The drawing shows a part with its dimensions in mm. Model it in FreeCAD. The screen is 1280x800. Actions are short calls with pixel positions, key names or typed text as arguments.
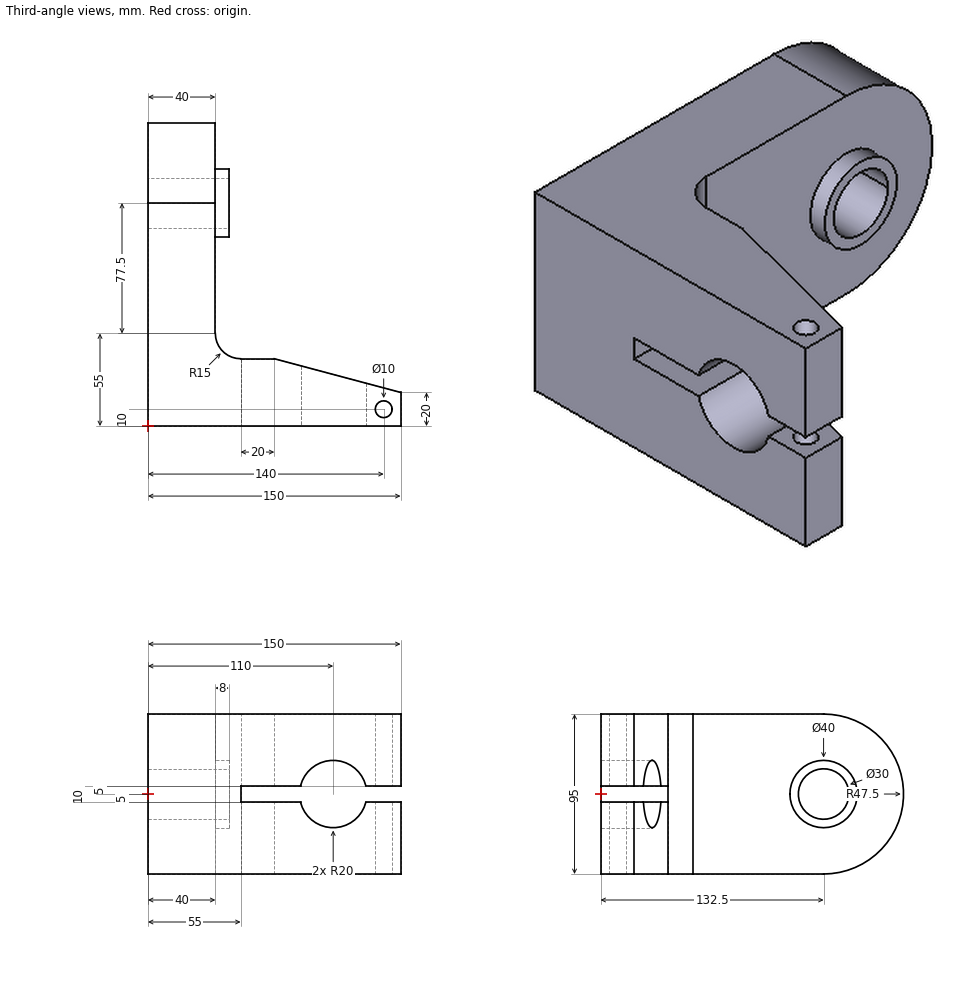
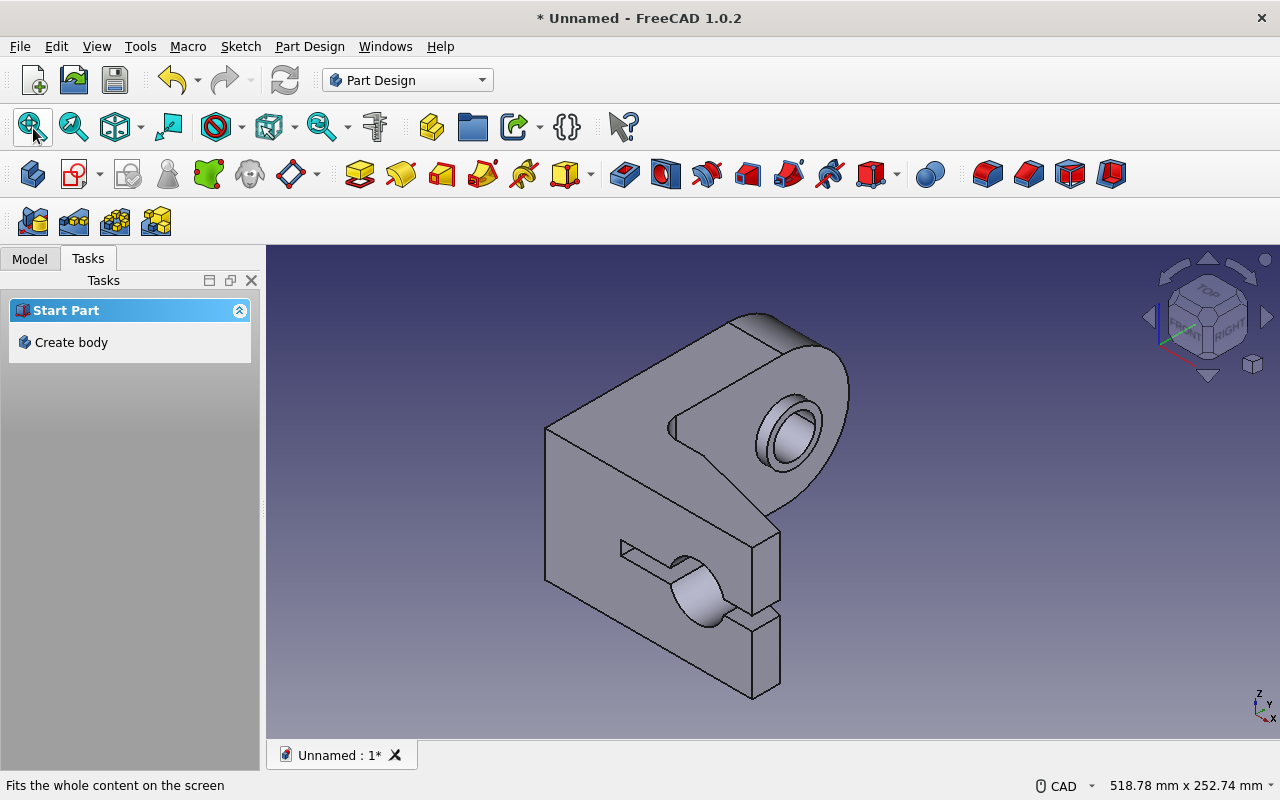
click(629, 430)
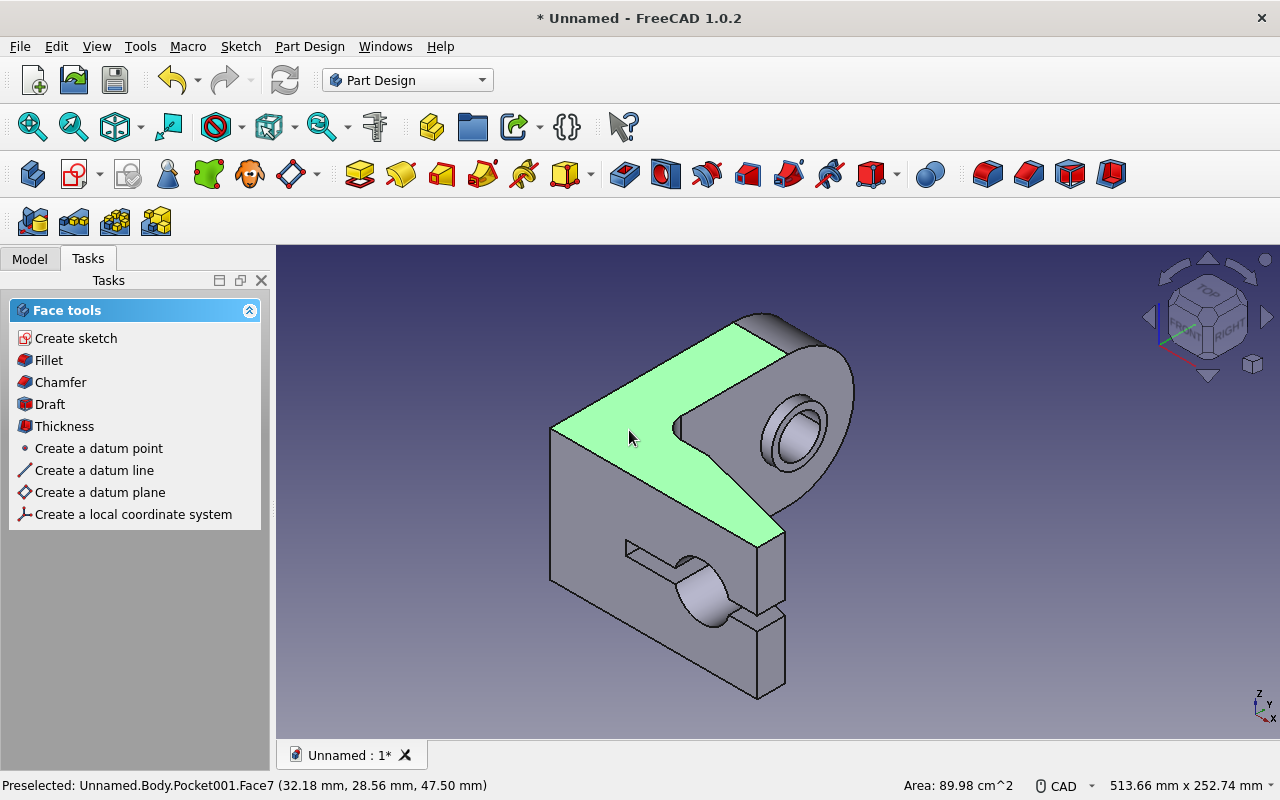
click(74, 174)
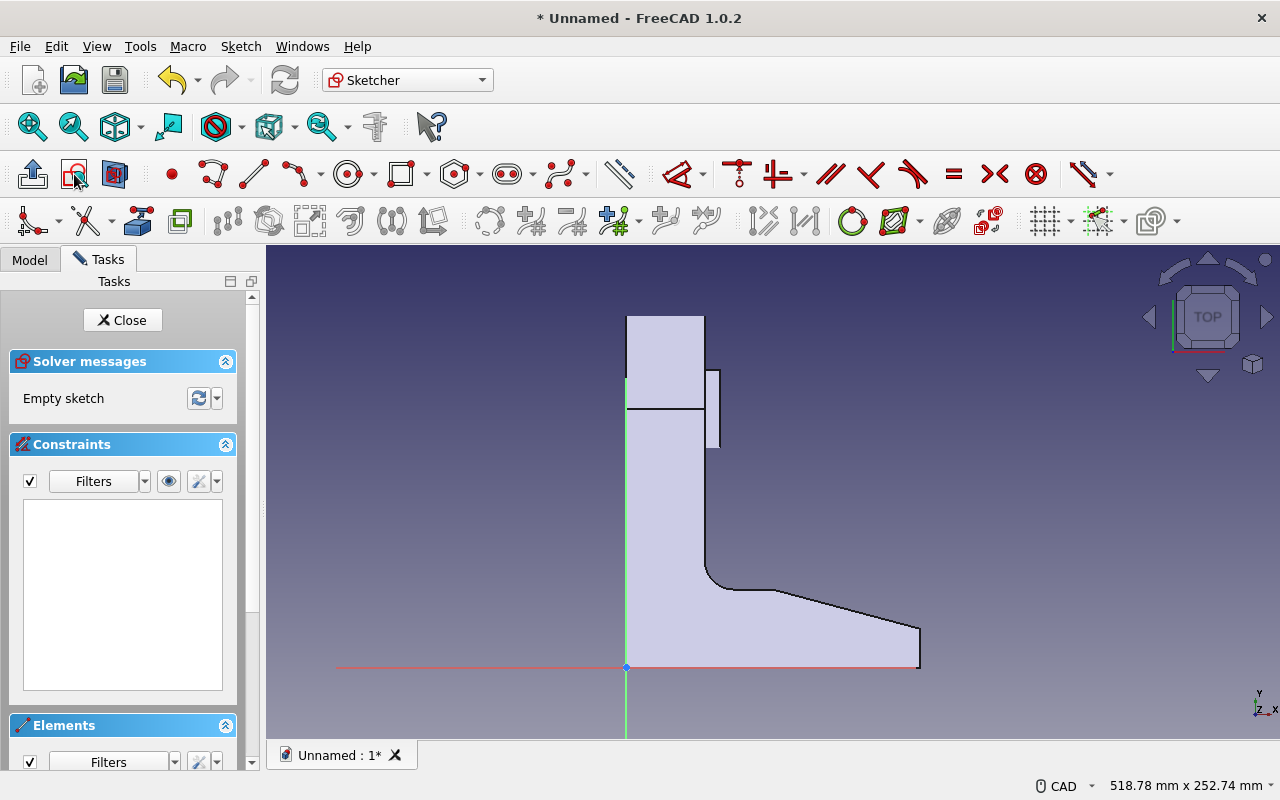
scroll(913, 658, up, 14)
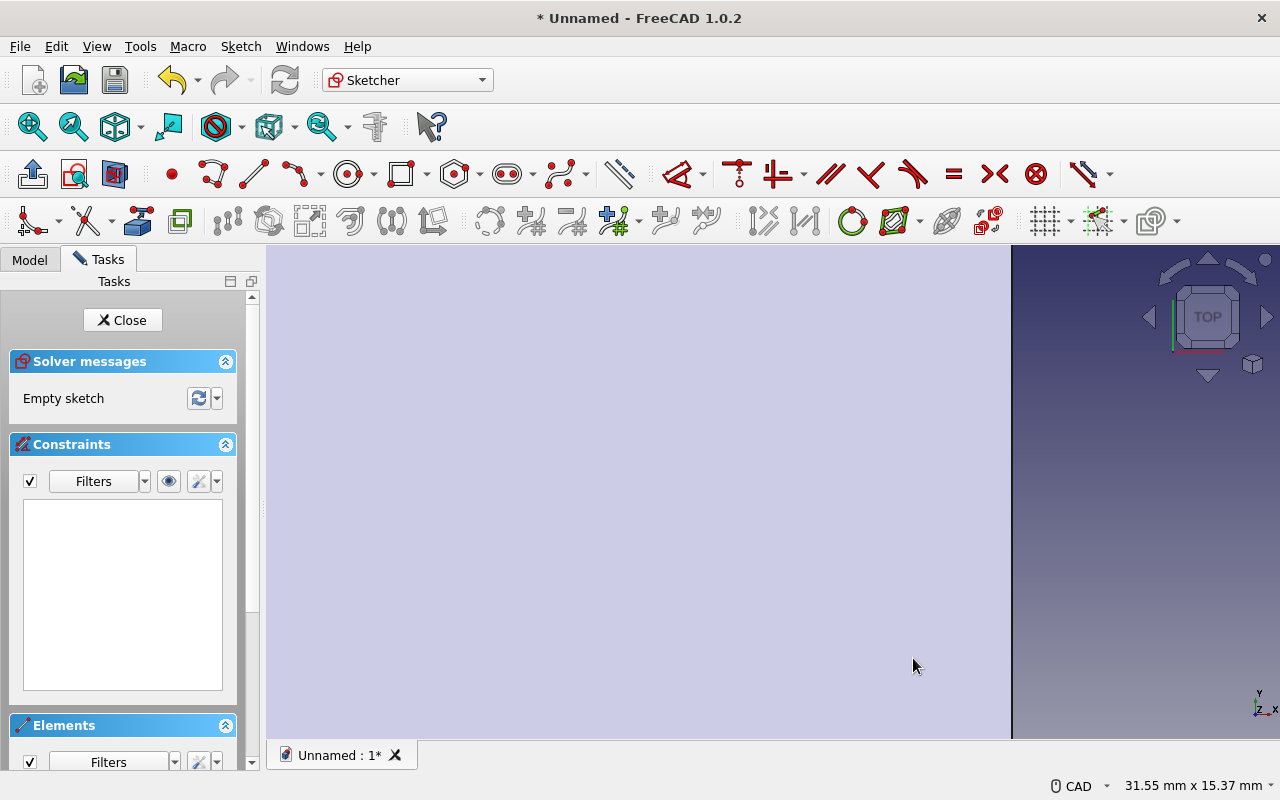
click(348, 174)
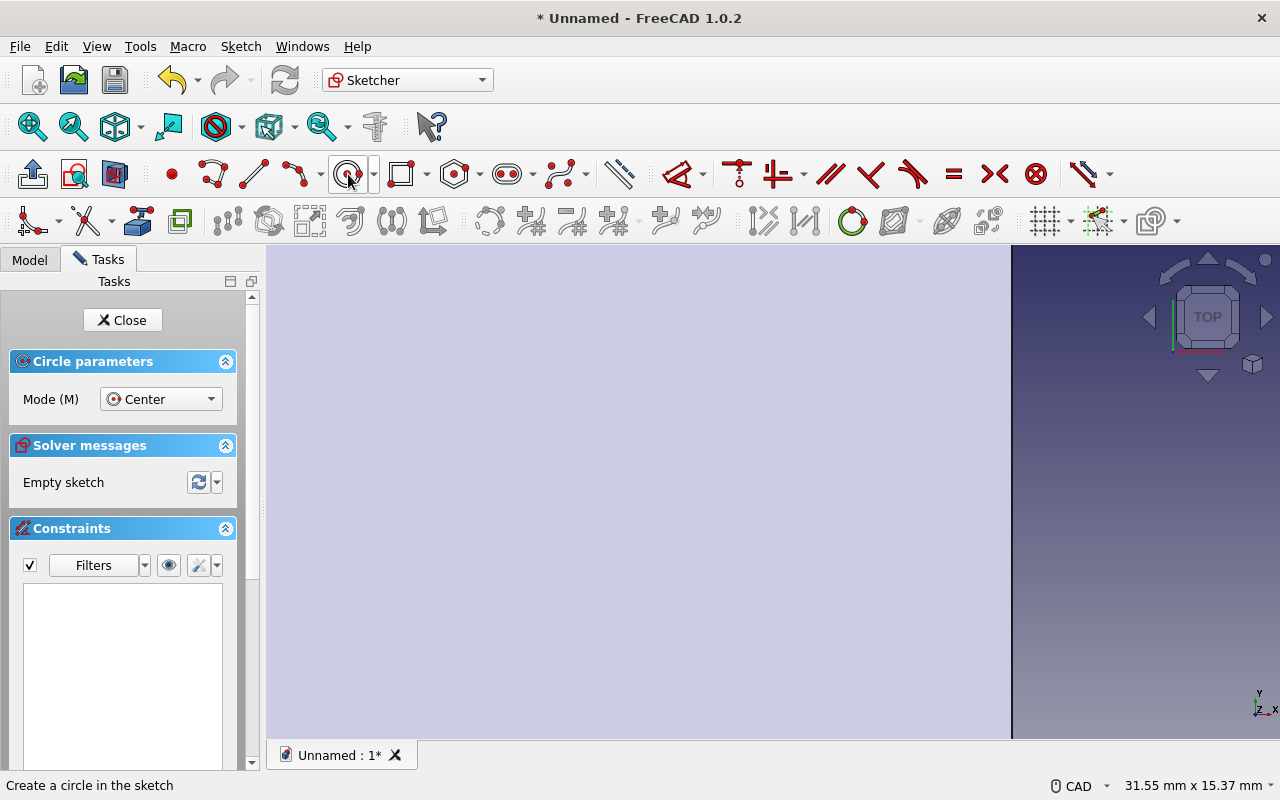
click(690, 485)
move(804, 371)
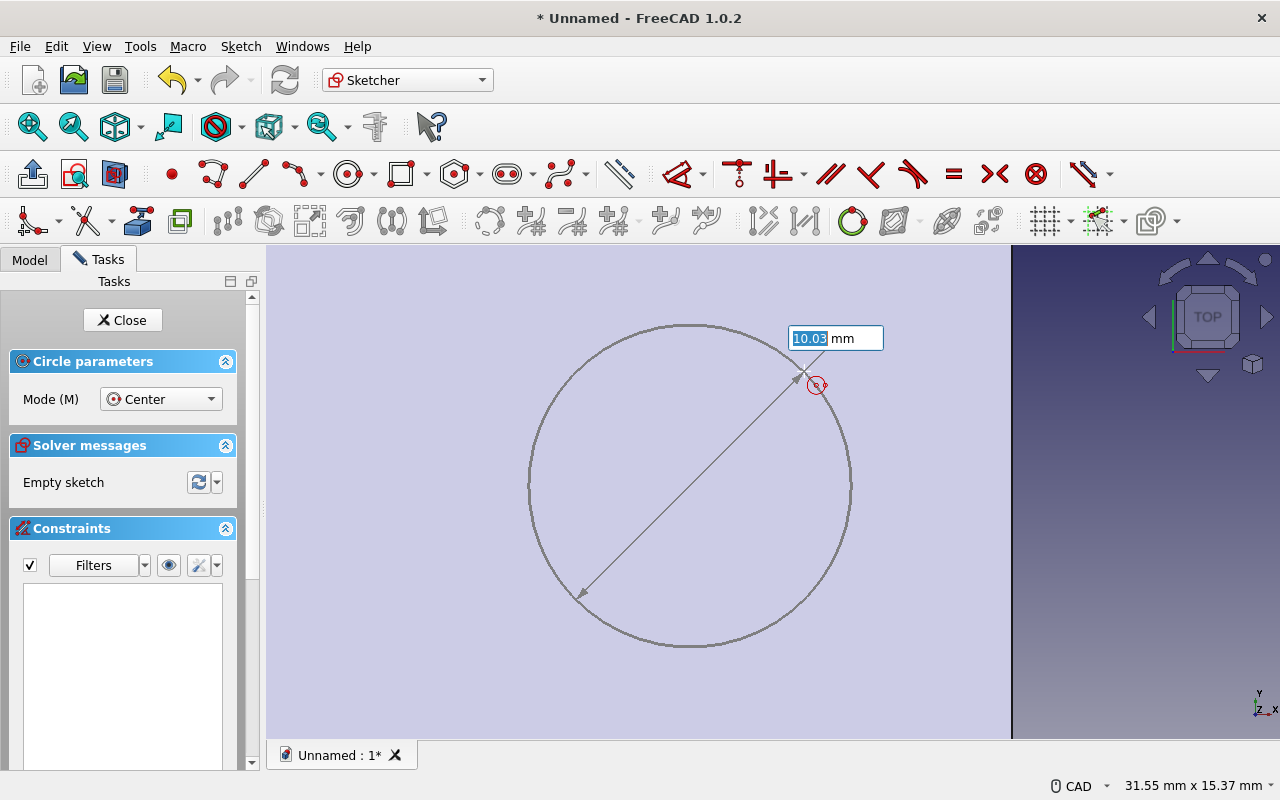
text(10)
key(Return)
key(Escape)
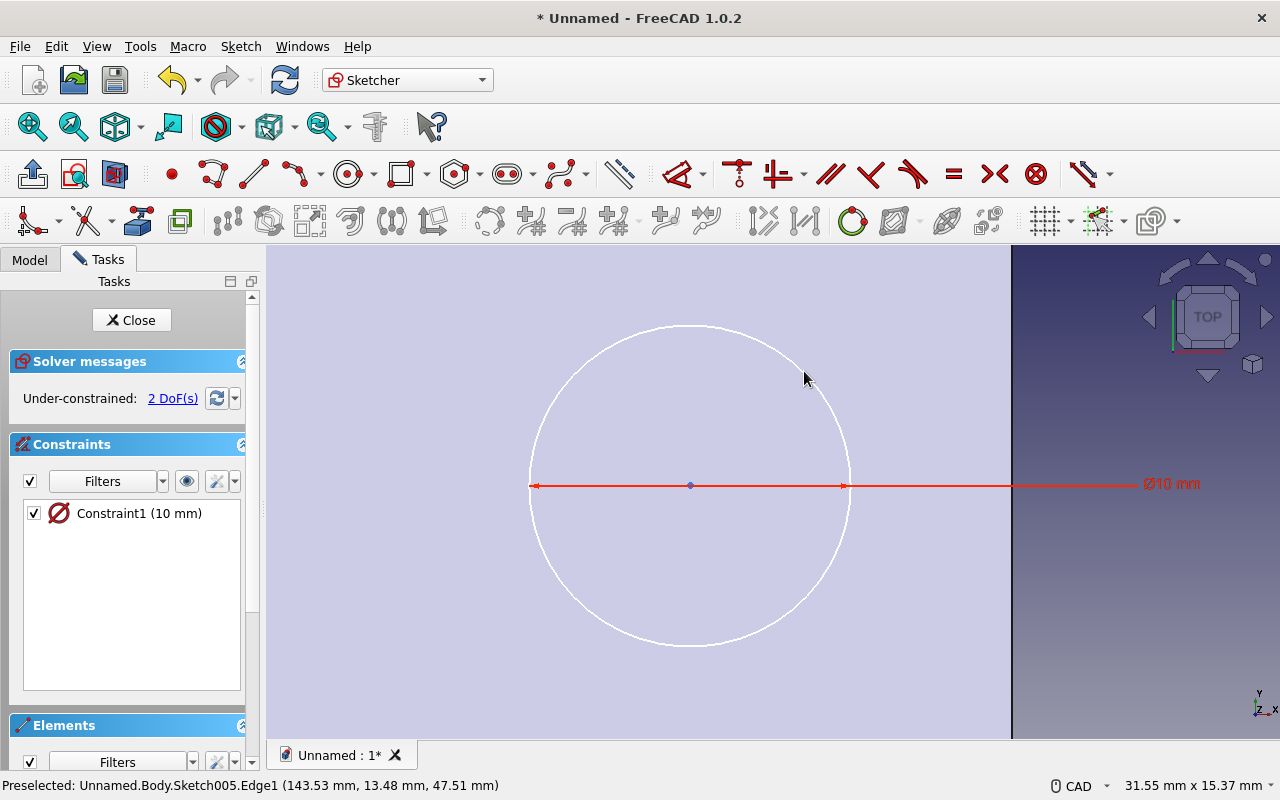
click(676, 174)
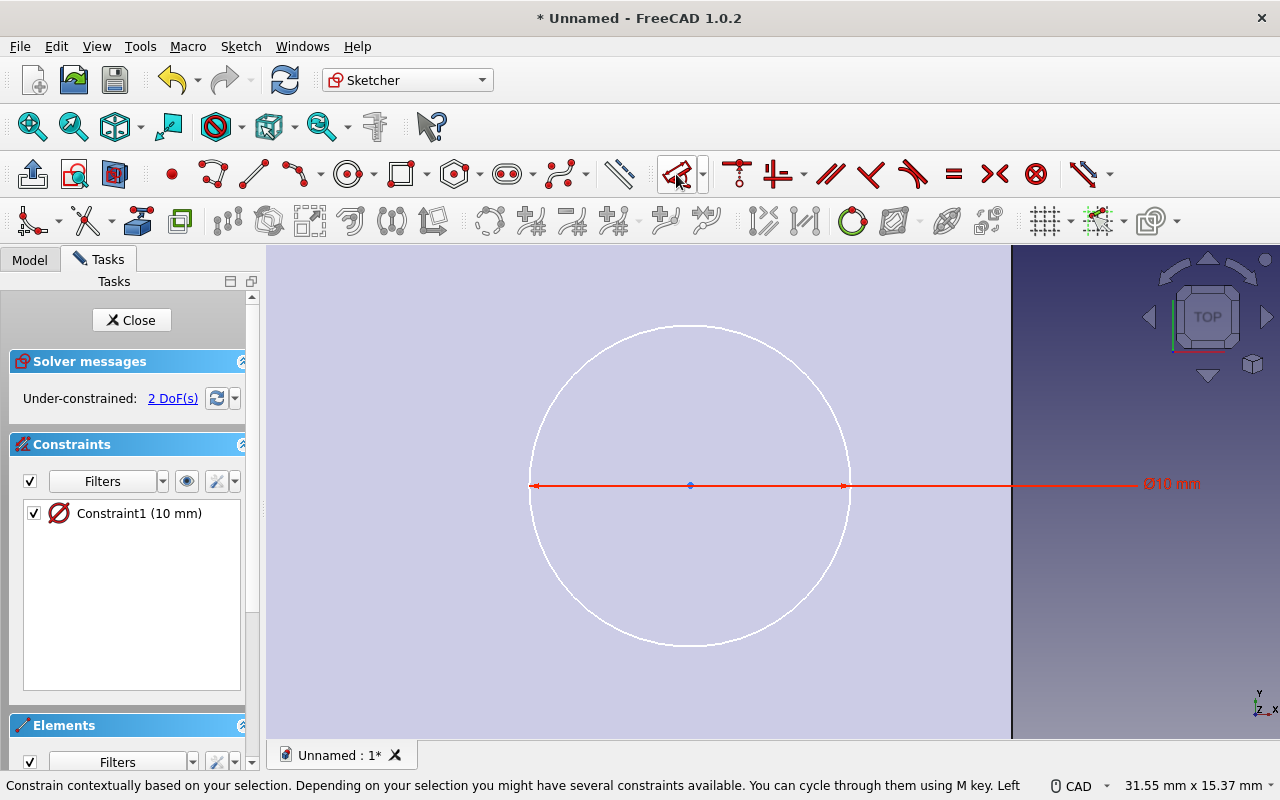
click(690, 486)
click(724, 598)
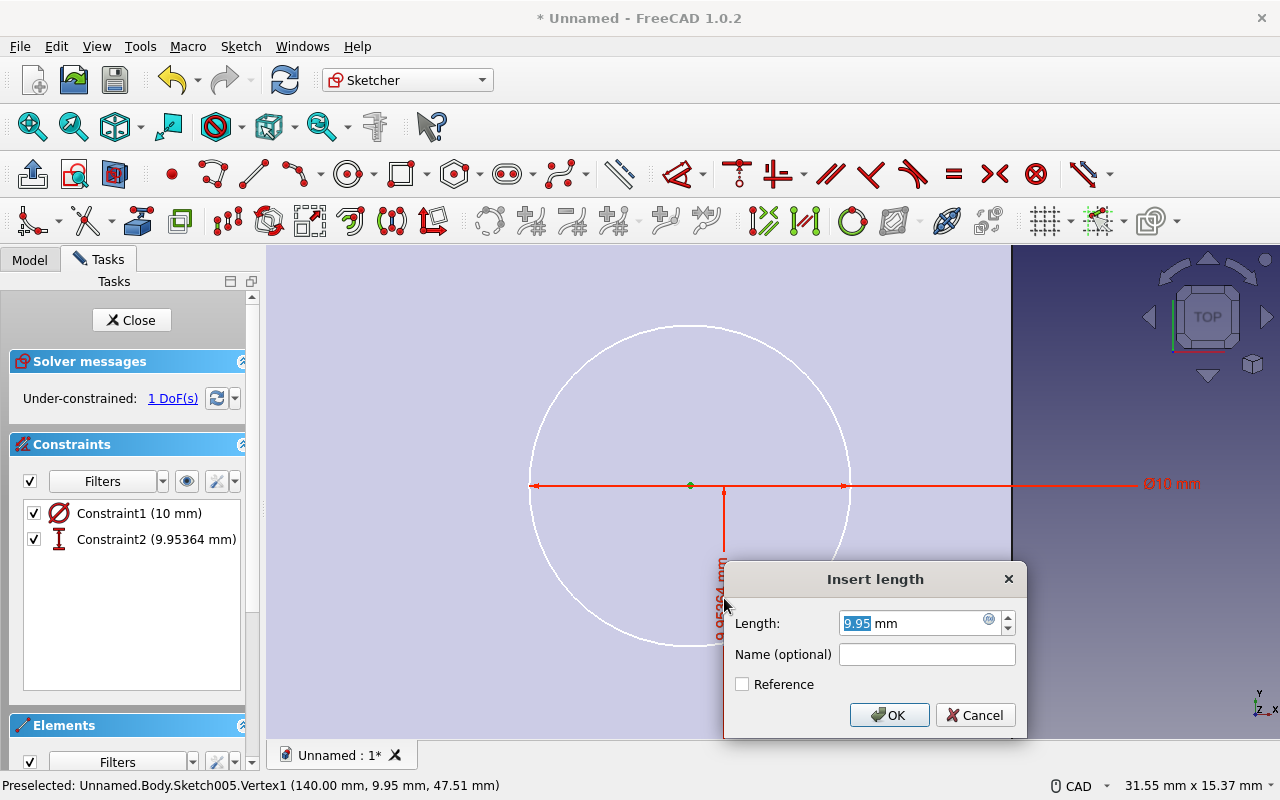
text(10)
key(Return)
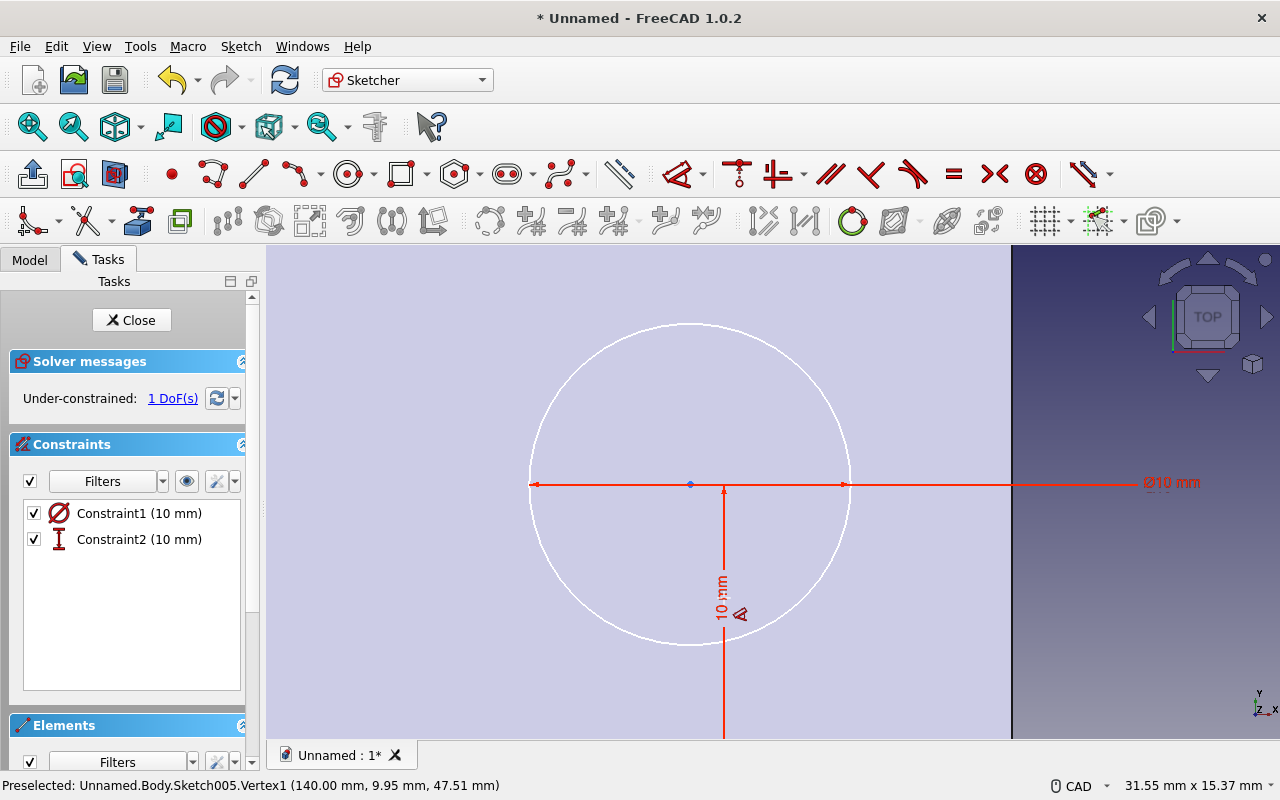
click(690, 485)
click(492, 451)